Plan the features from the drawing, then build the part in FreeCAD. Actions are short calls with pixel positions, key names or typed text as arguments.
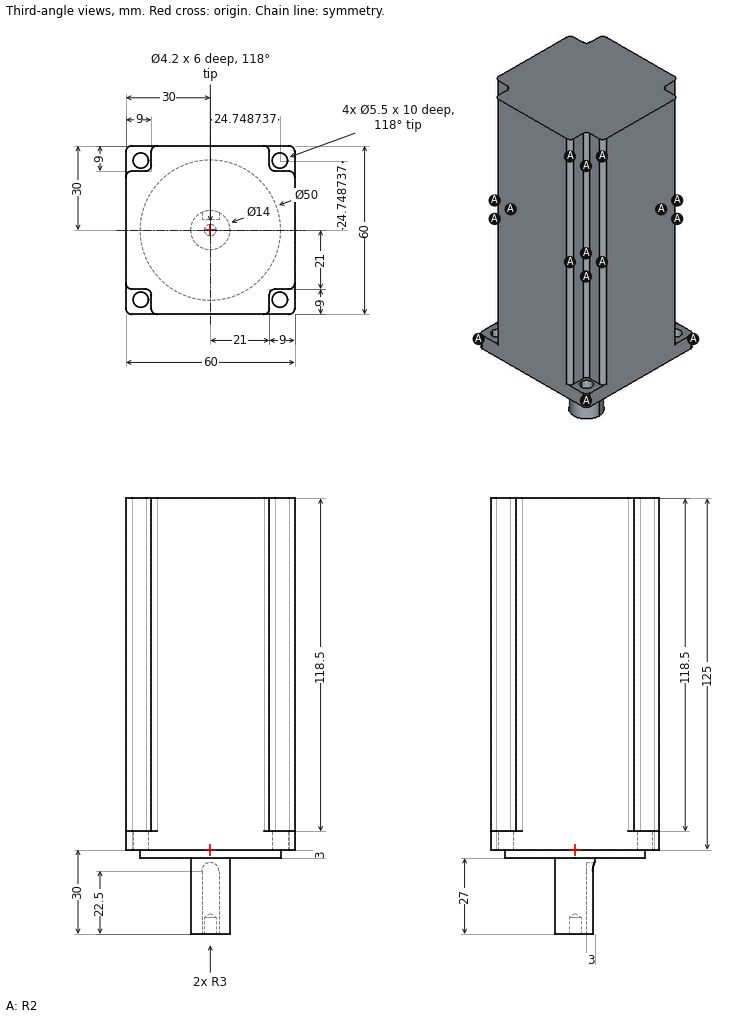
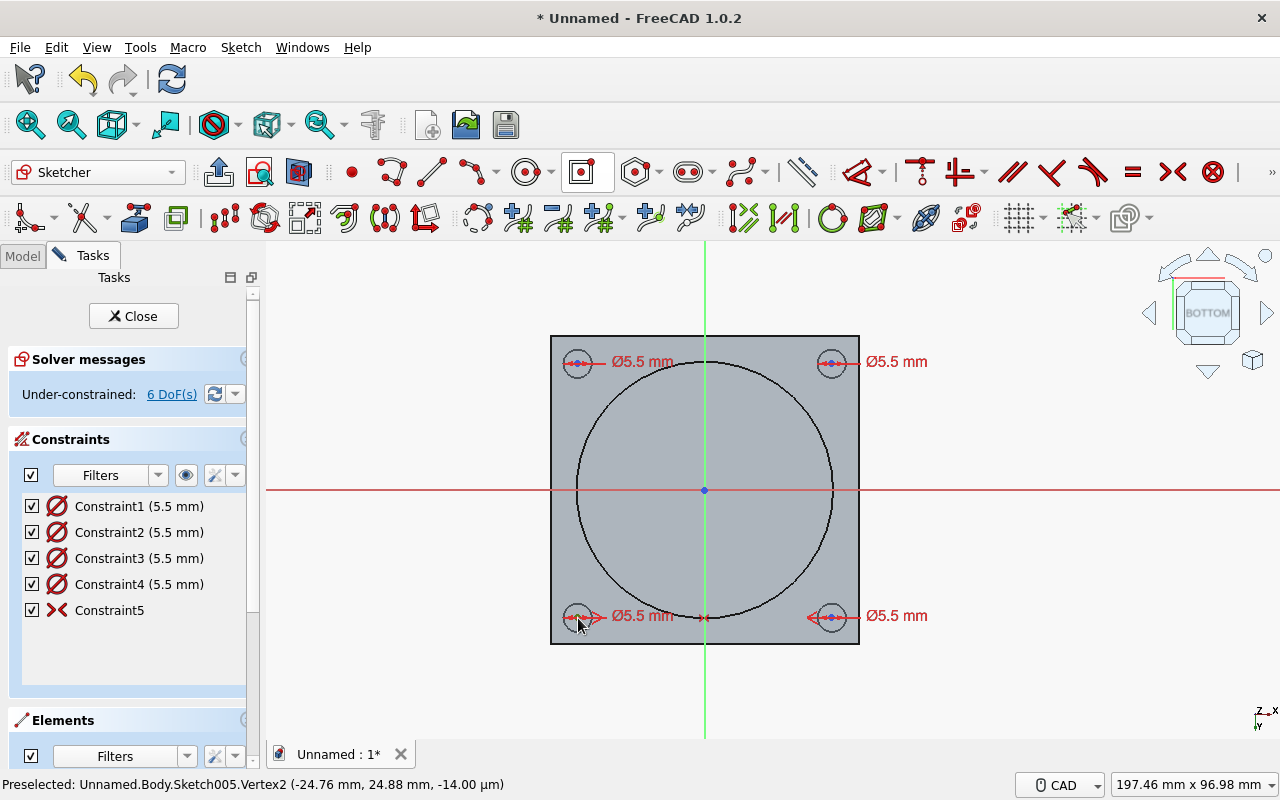
click(578, 364)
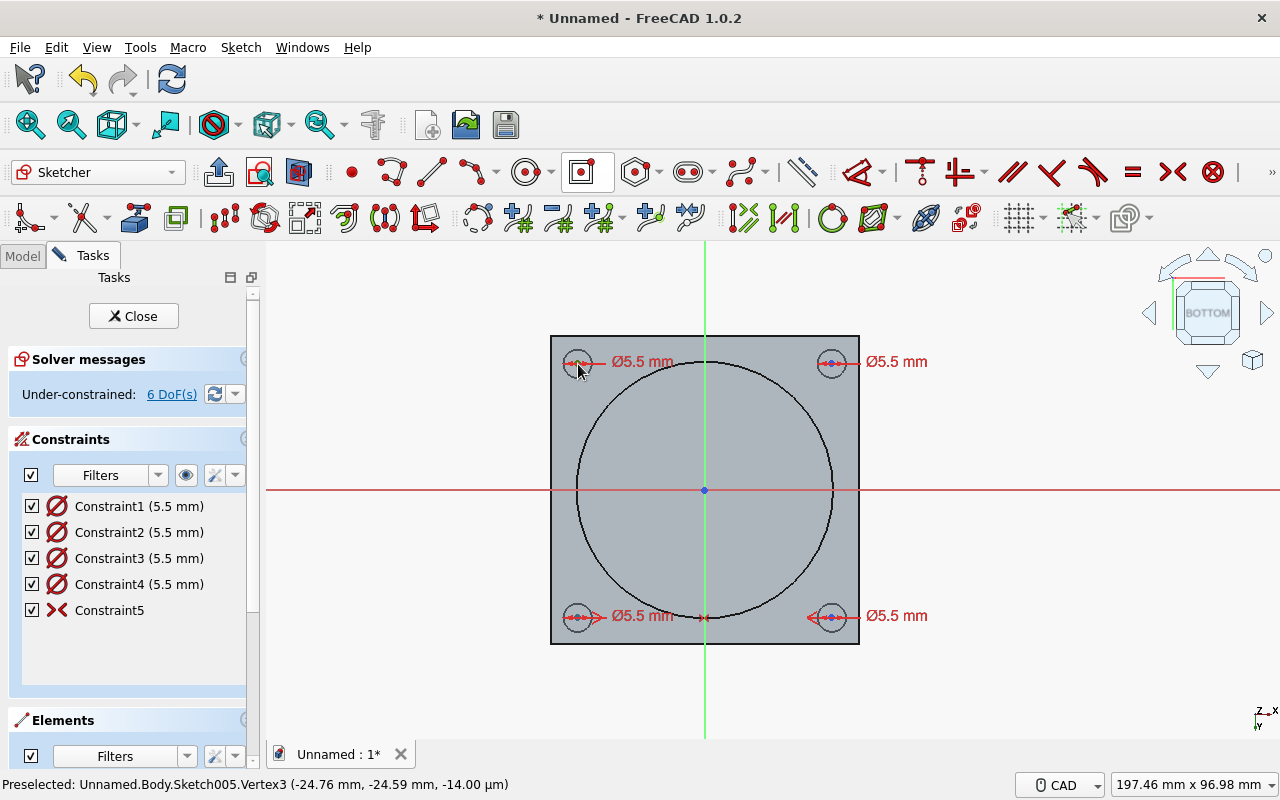
click(353, 490)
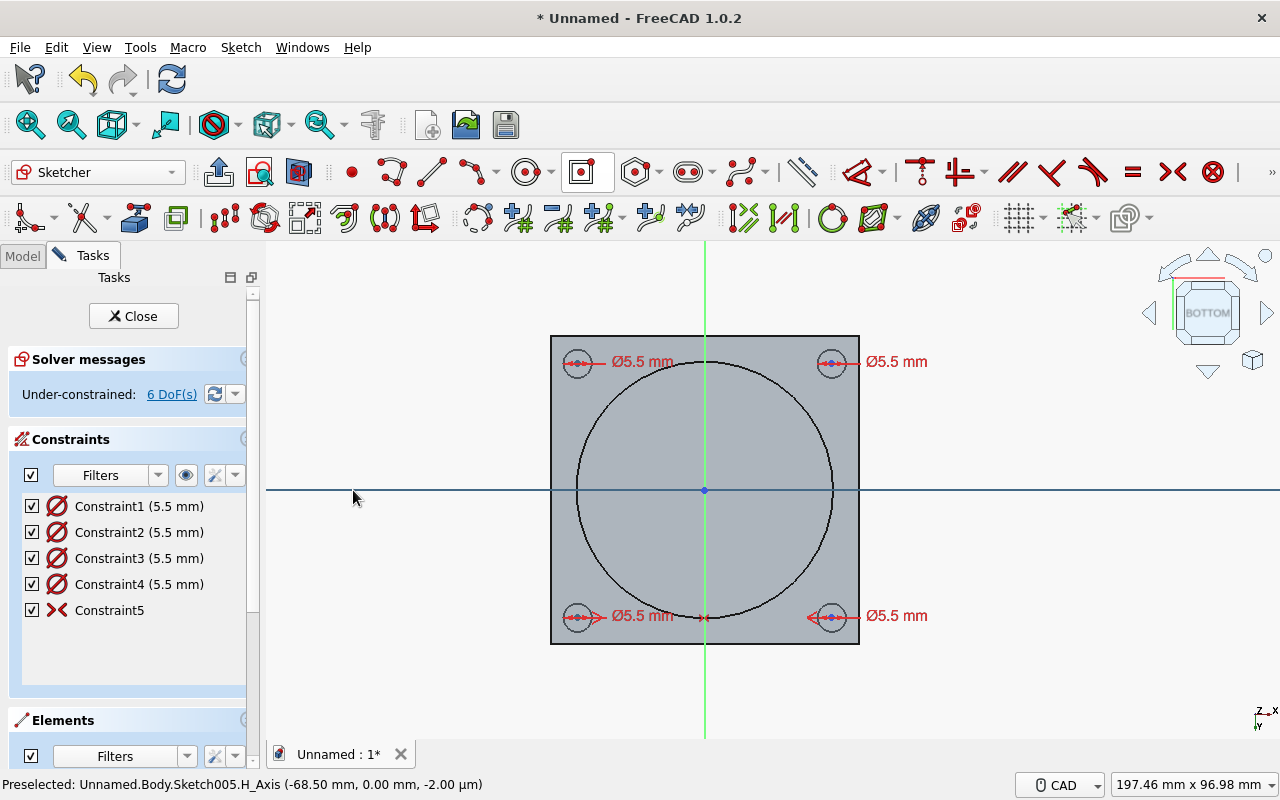
click(1174, 172)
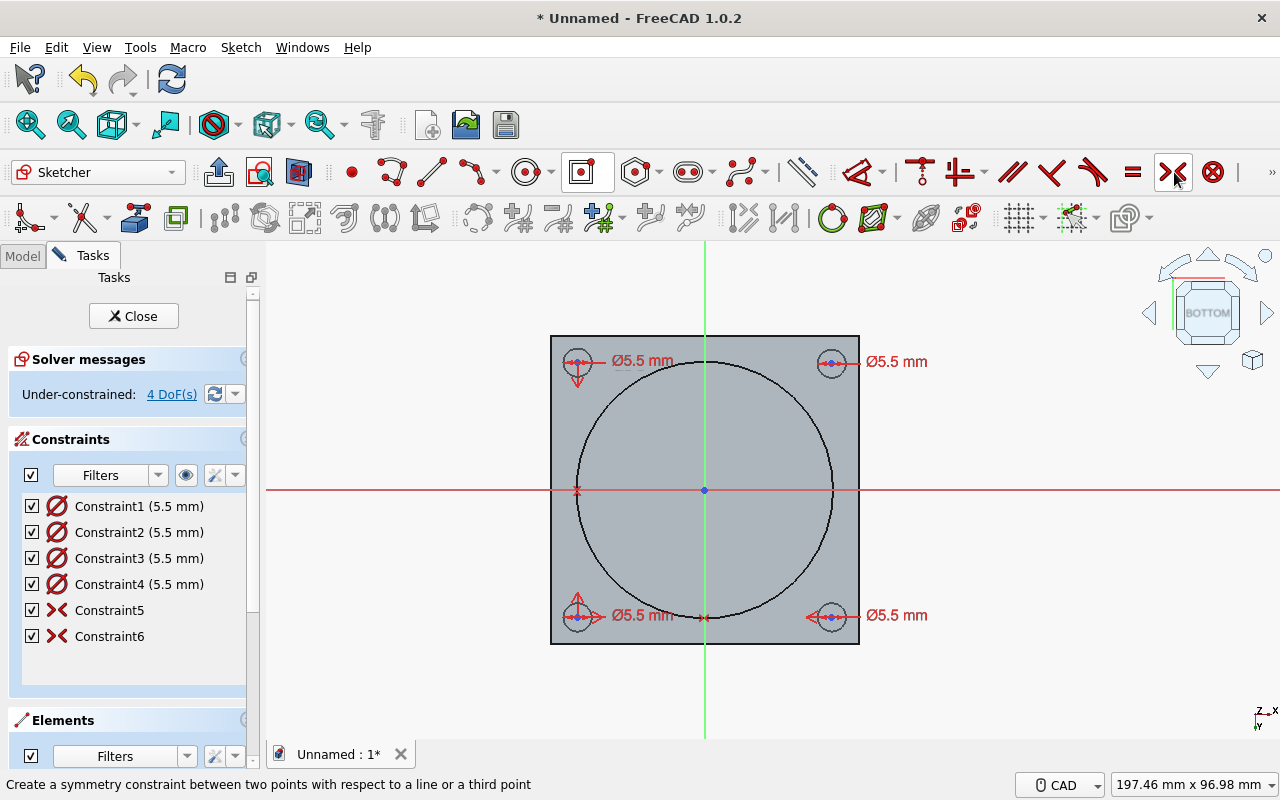
click(832, 617)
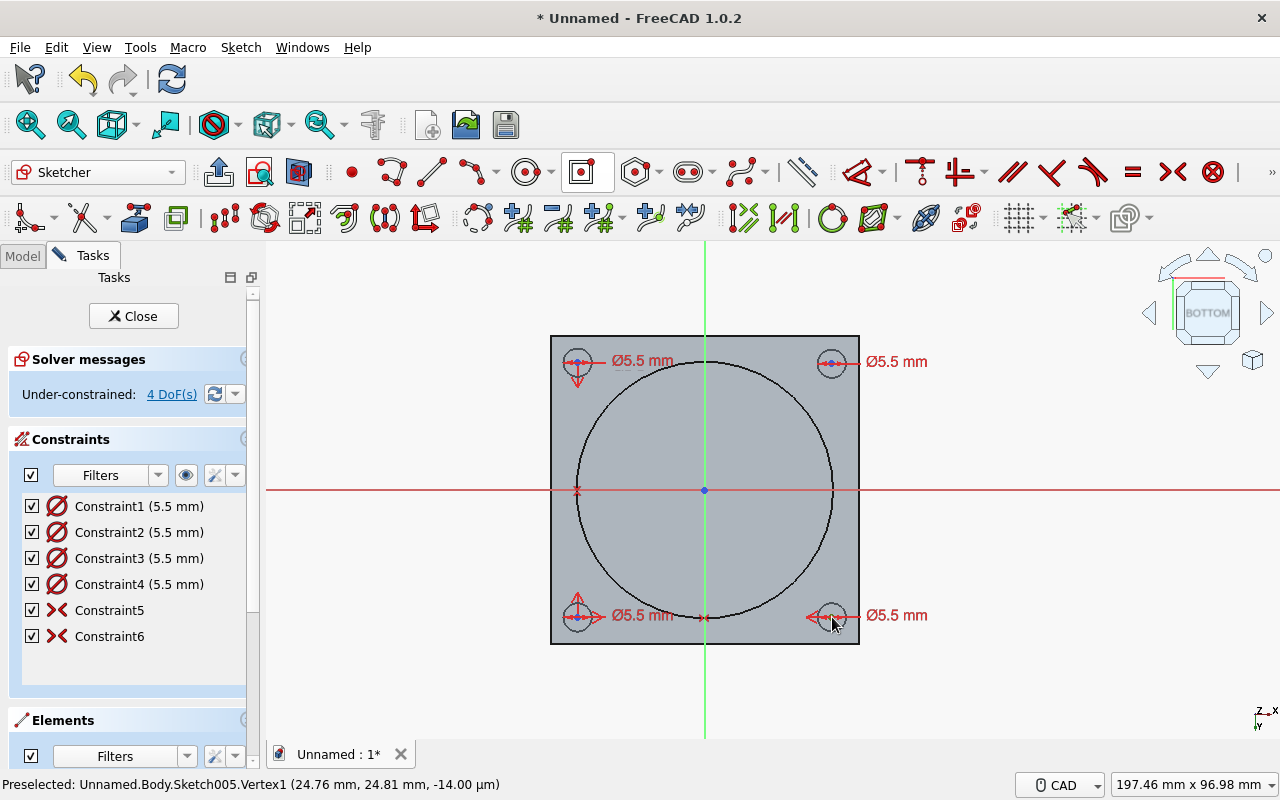
click(832, 364)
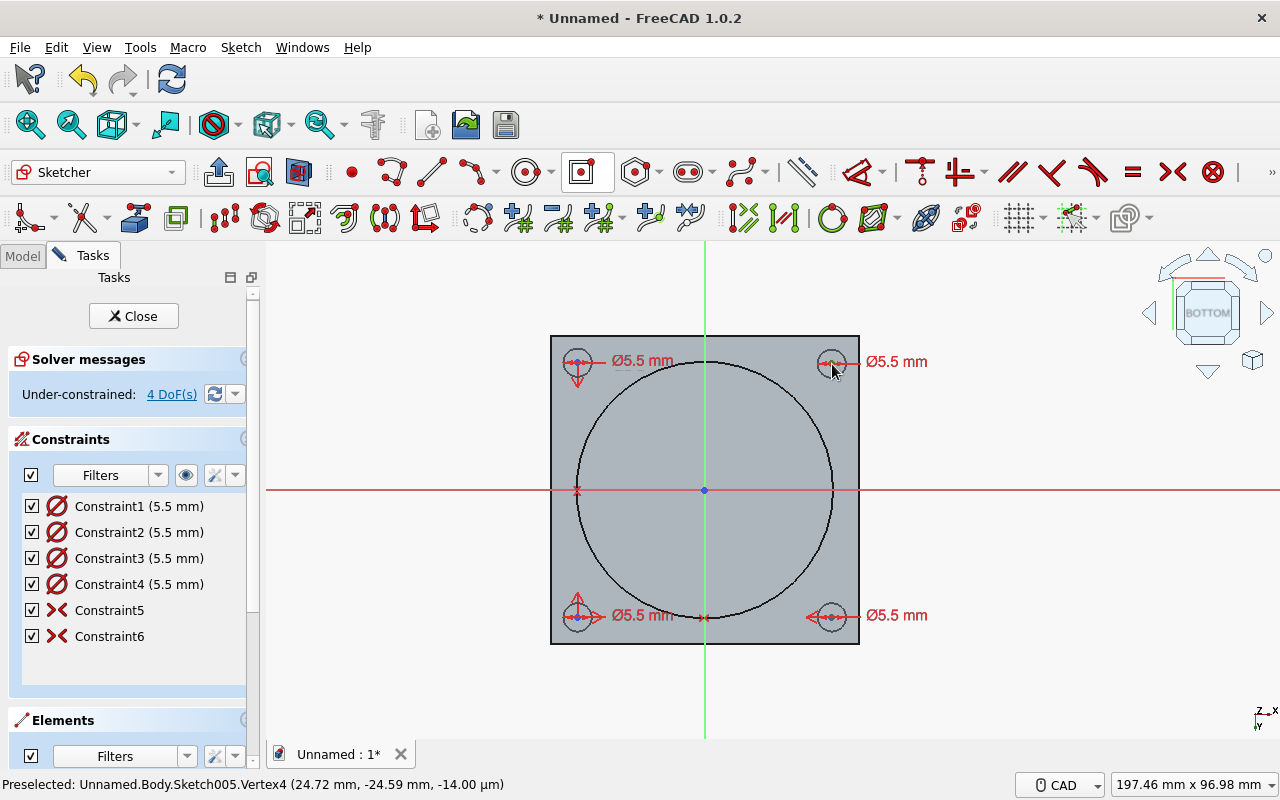
click(353, 490)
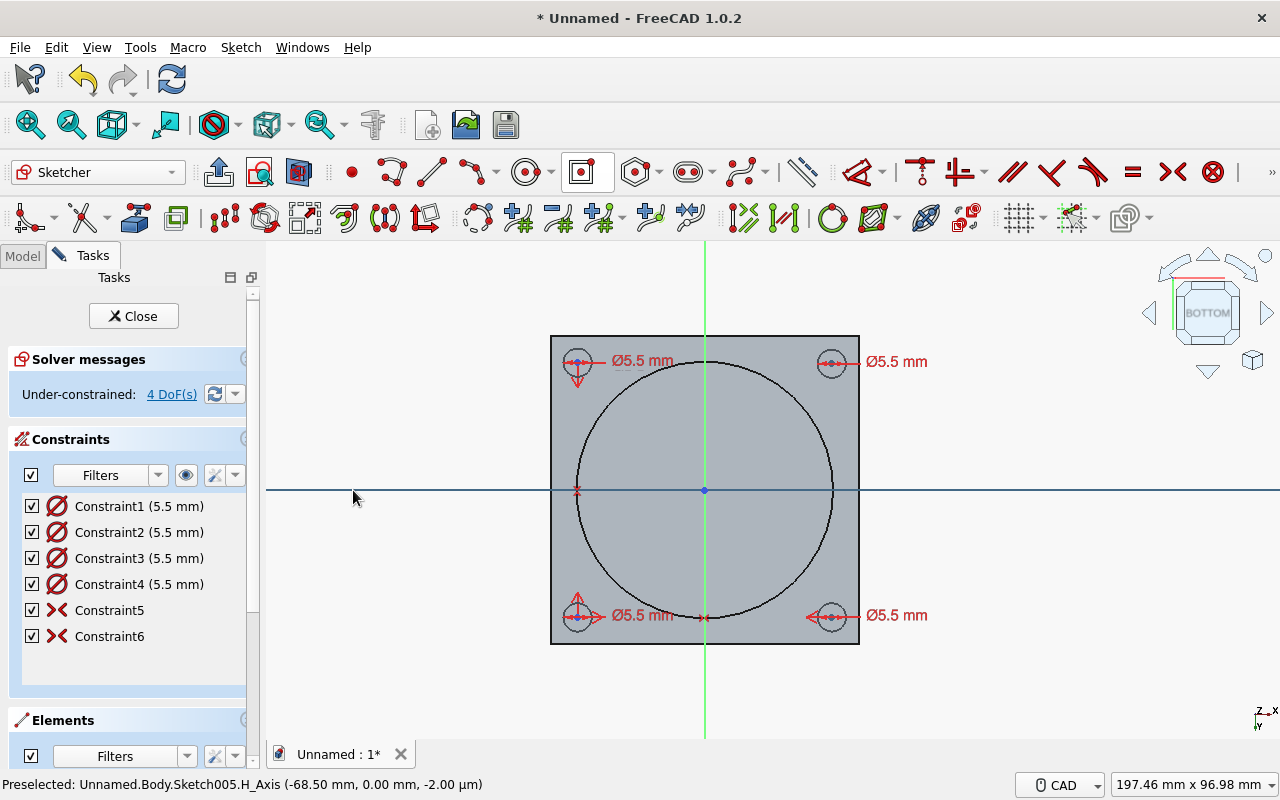
click(1174, 172)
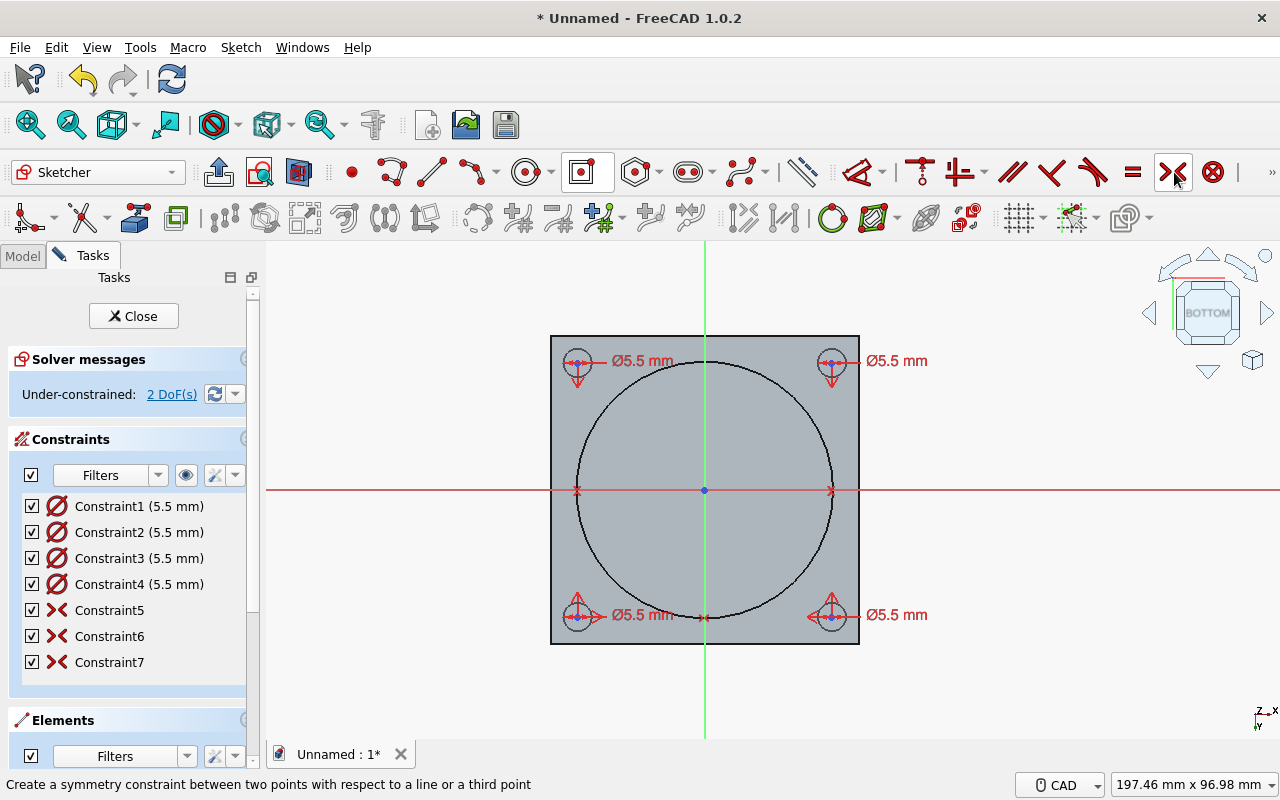
click(858, 172)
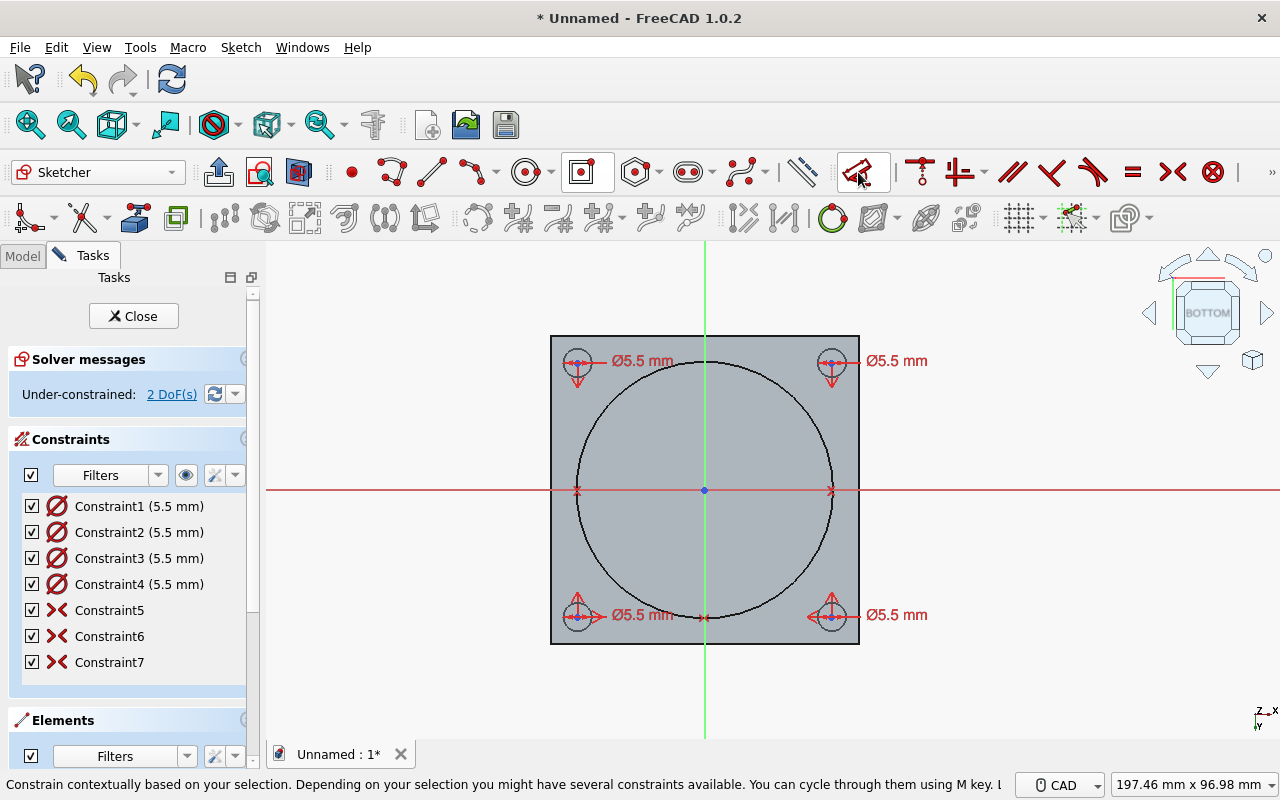
click(832, 617)
click(768, 651)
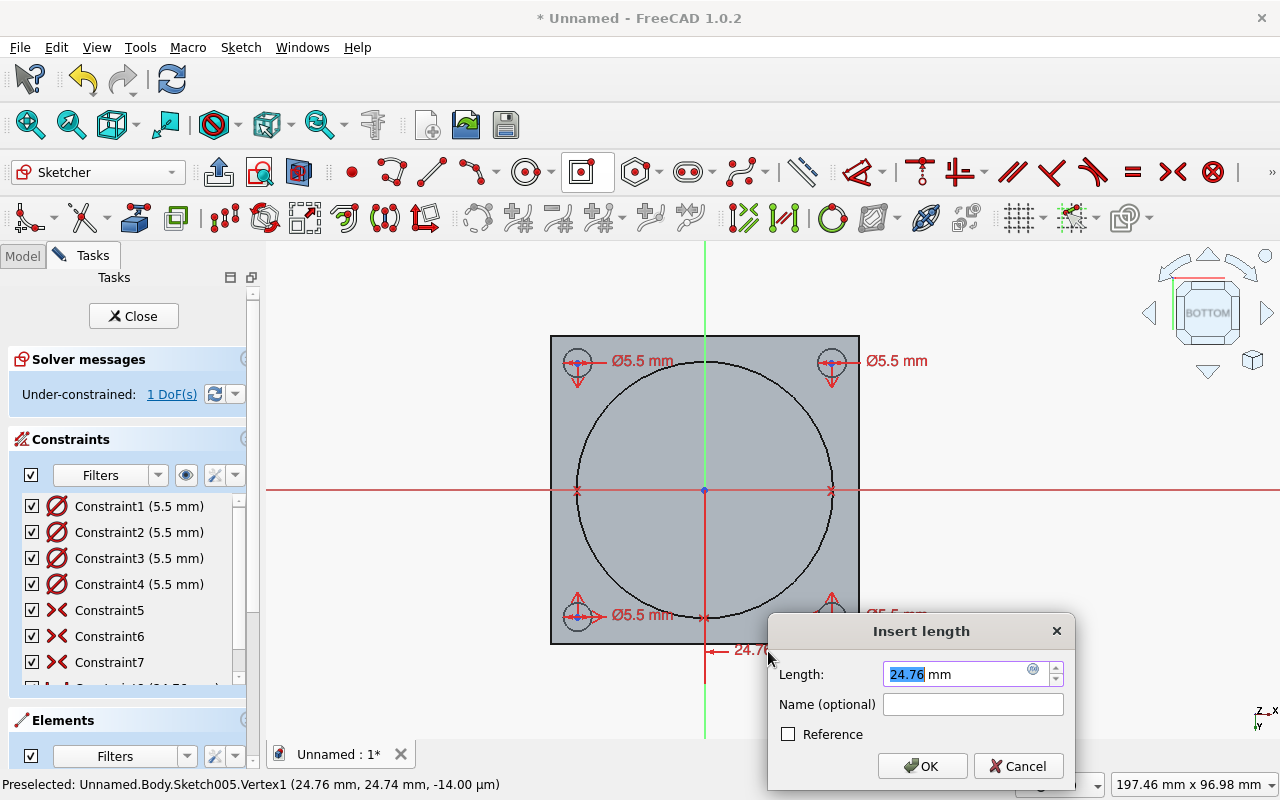
text(24.748737)
key(Return)